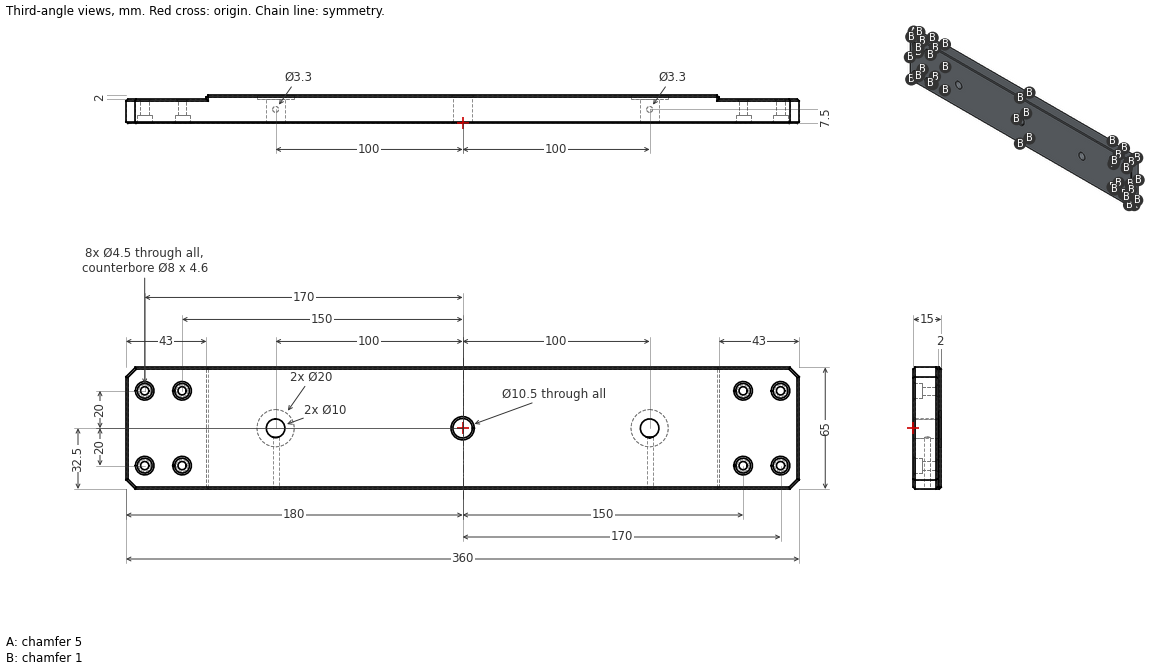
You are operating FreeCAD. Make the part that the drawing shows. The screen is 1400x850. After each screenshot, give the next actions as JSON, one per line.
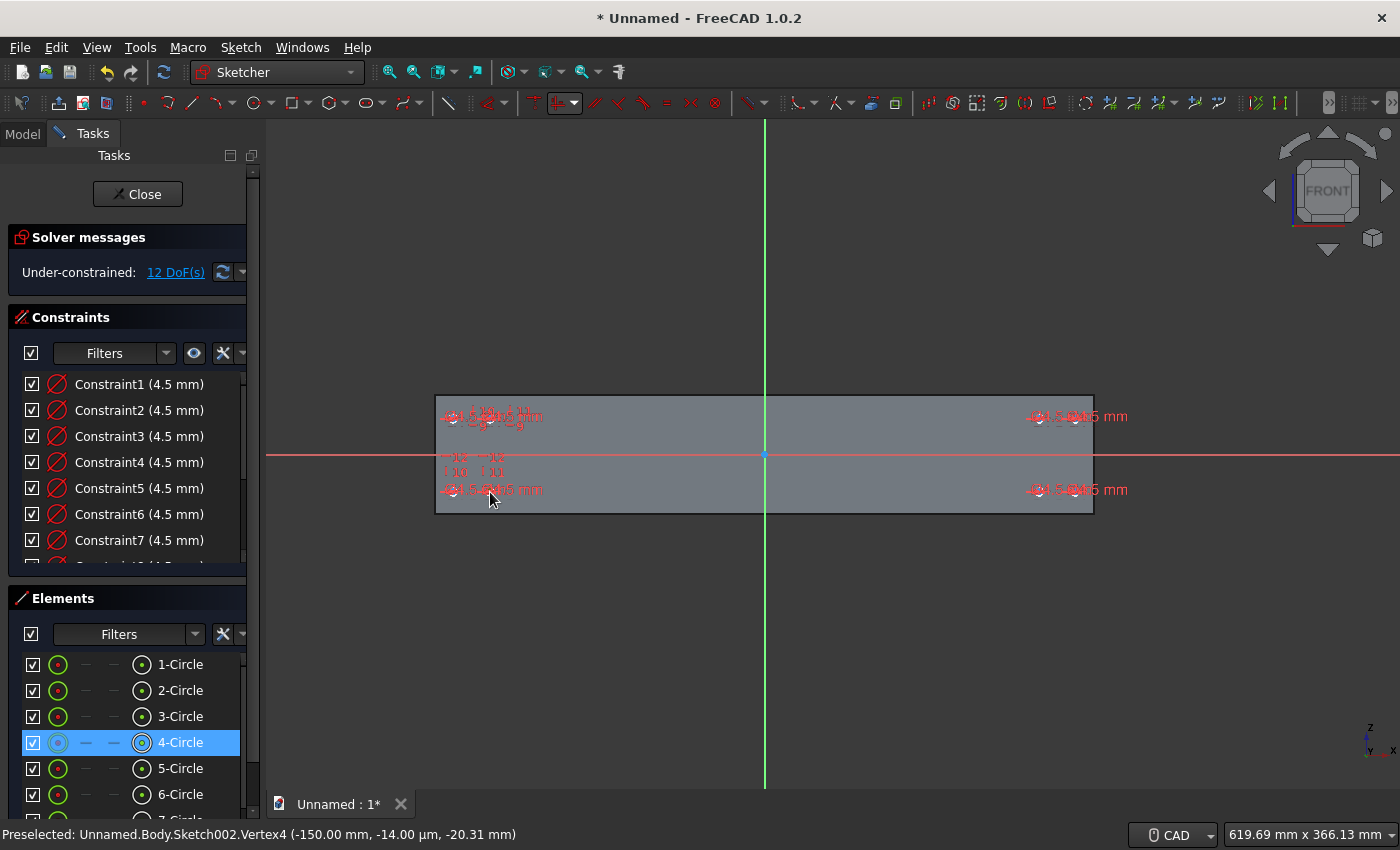
{"action": "left_click", "coordinate": [1039, 492]}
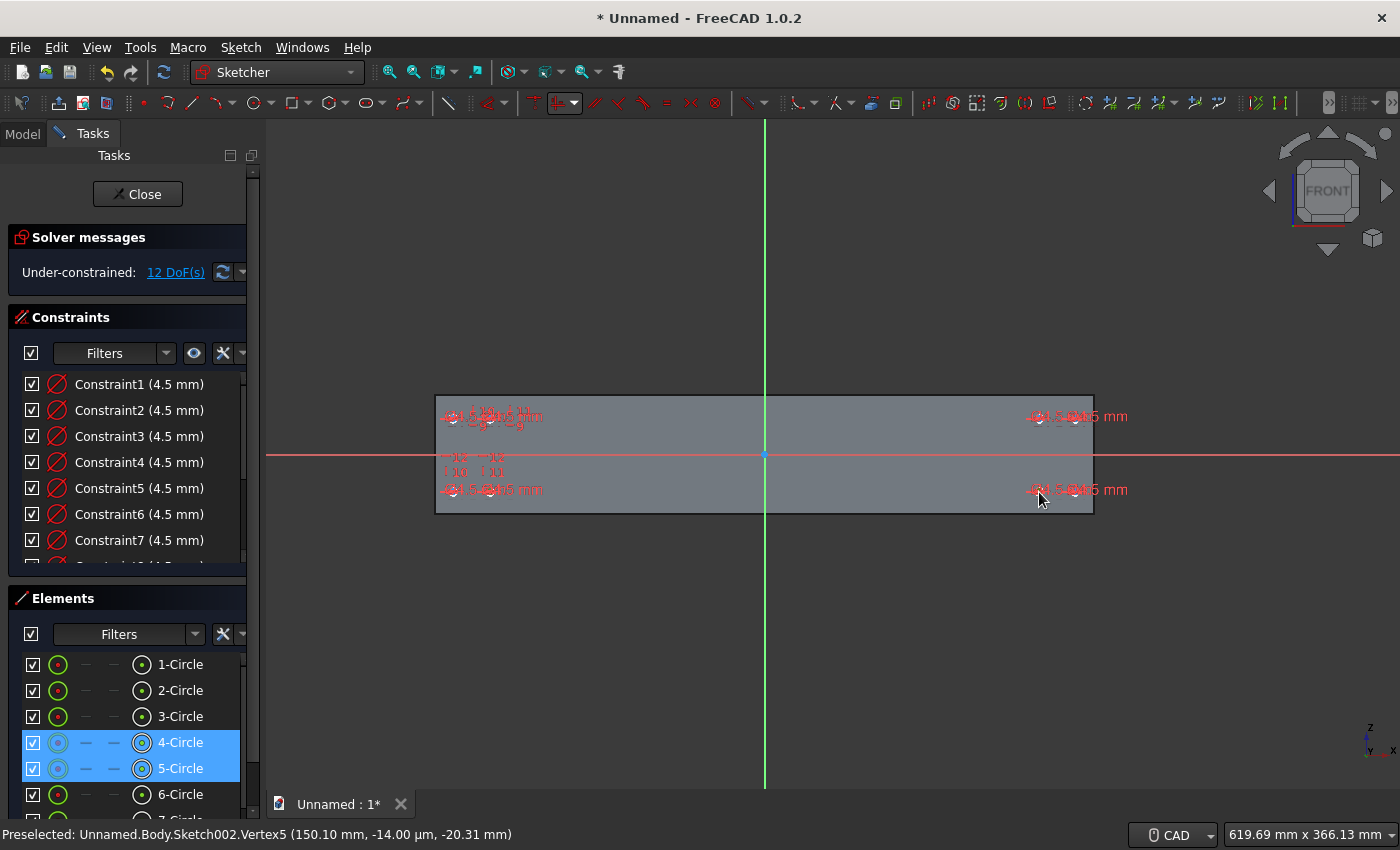
{"action": "left_click", "coordinate": [576, 104]}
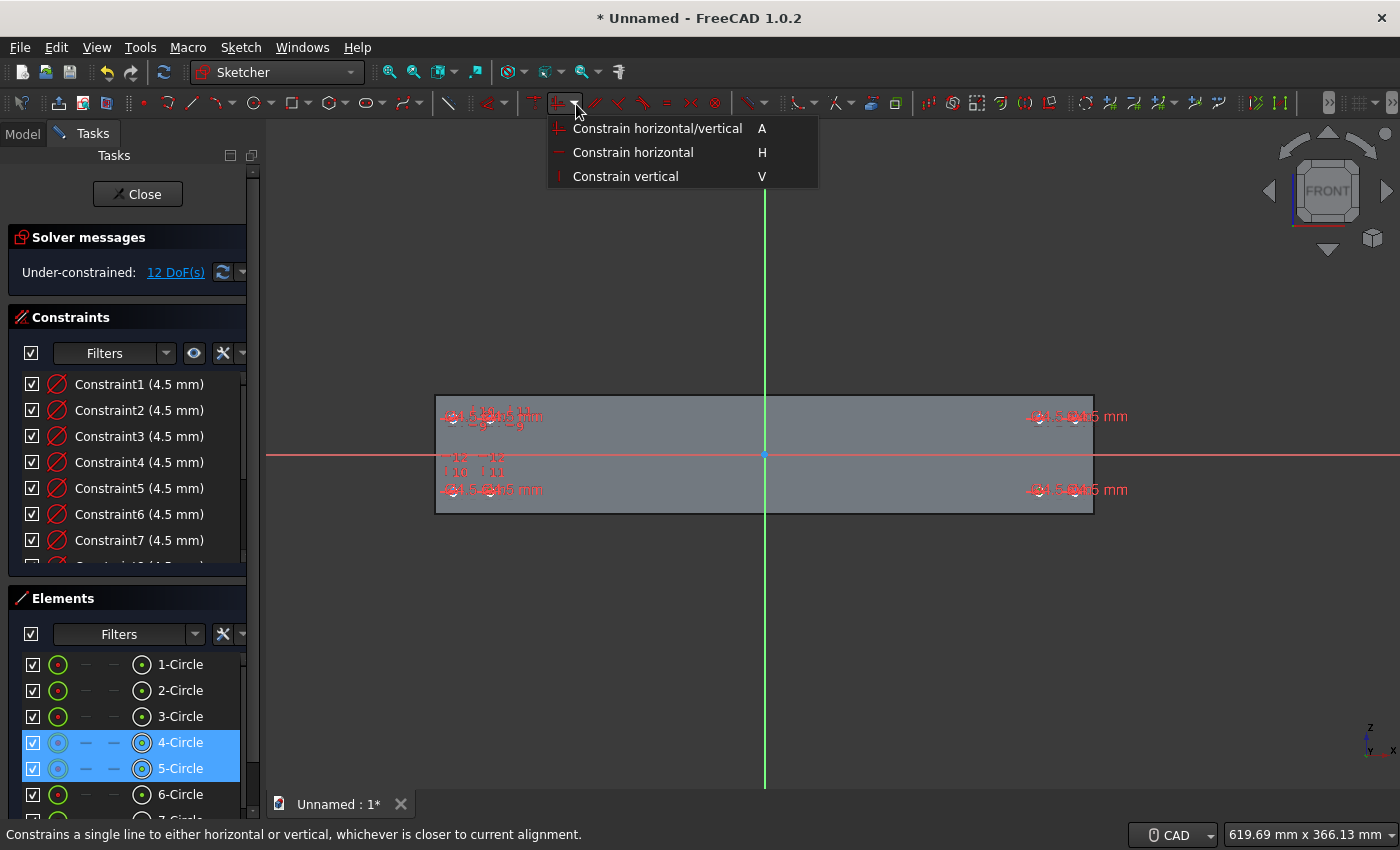
{"action": "left_click", "coordinate": [683, 152]}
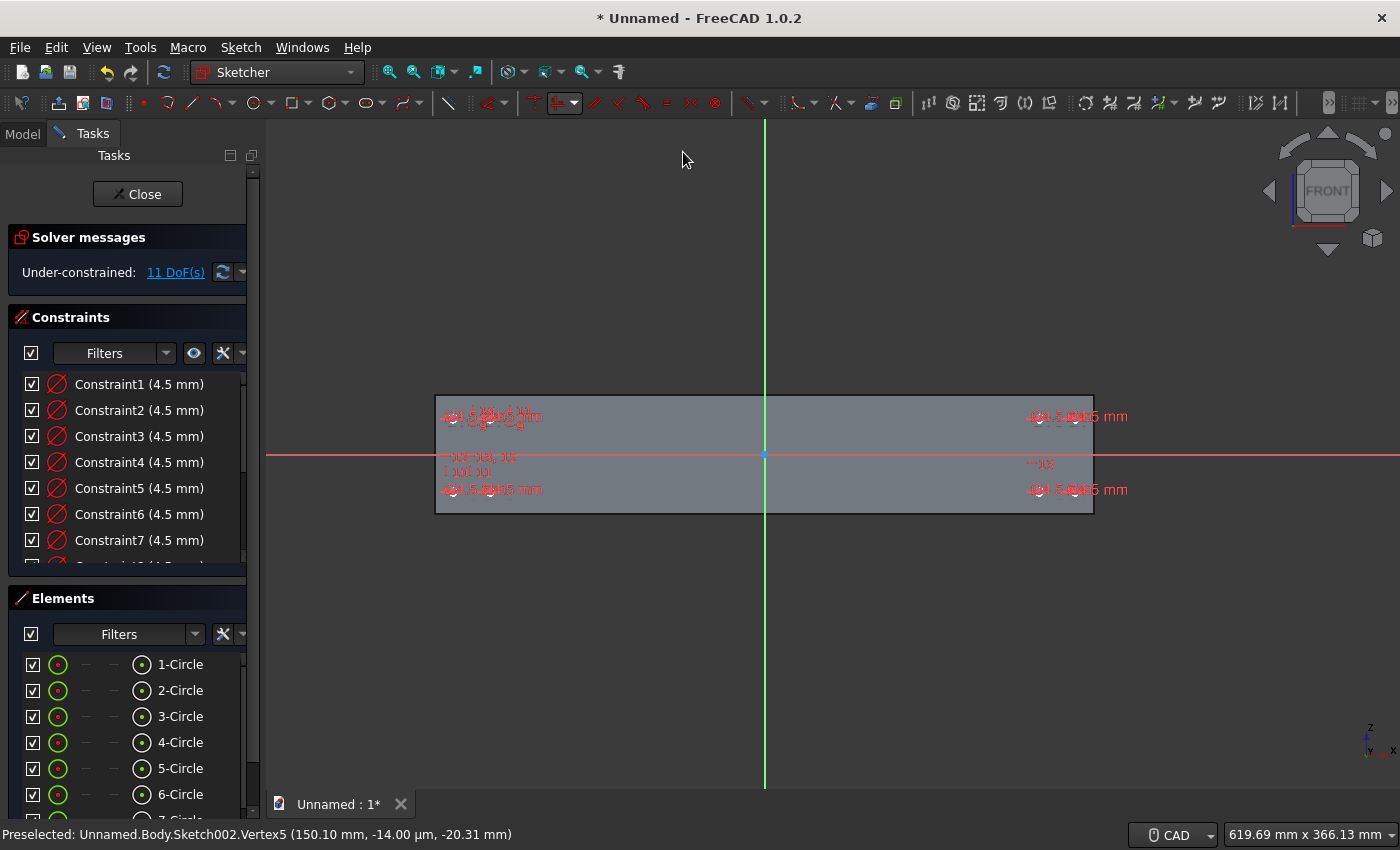
{"action": "left_click", "coordinate": [1039, 492]}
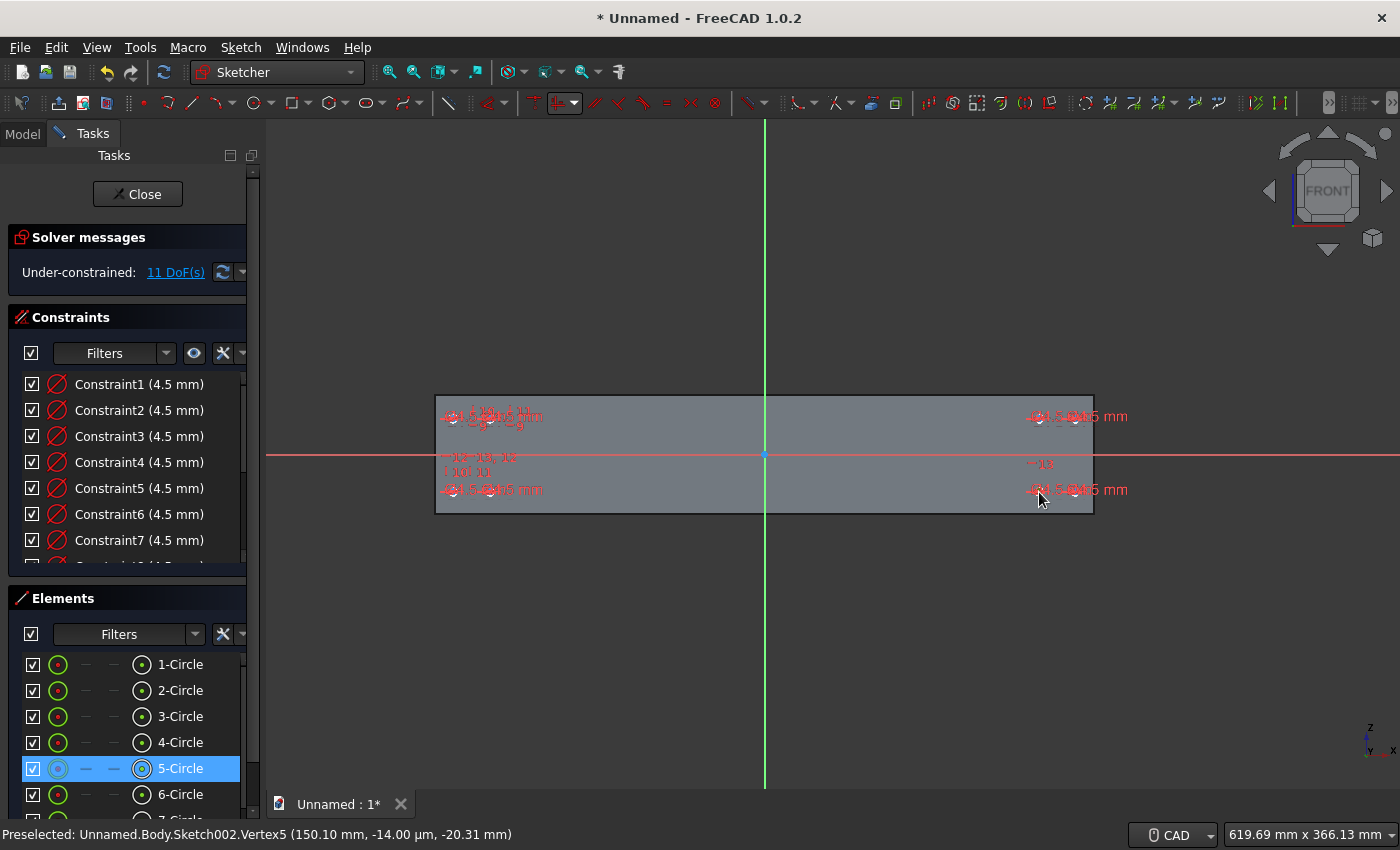
{"action": "left_click", "coordinate": [1075, 492]}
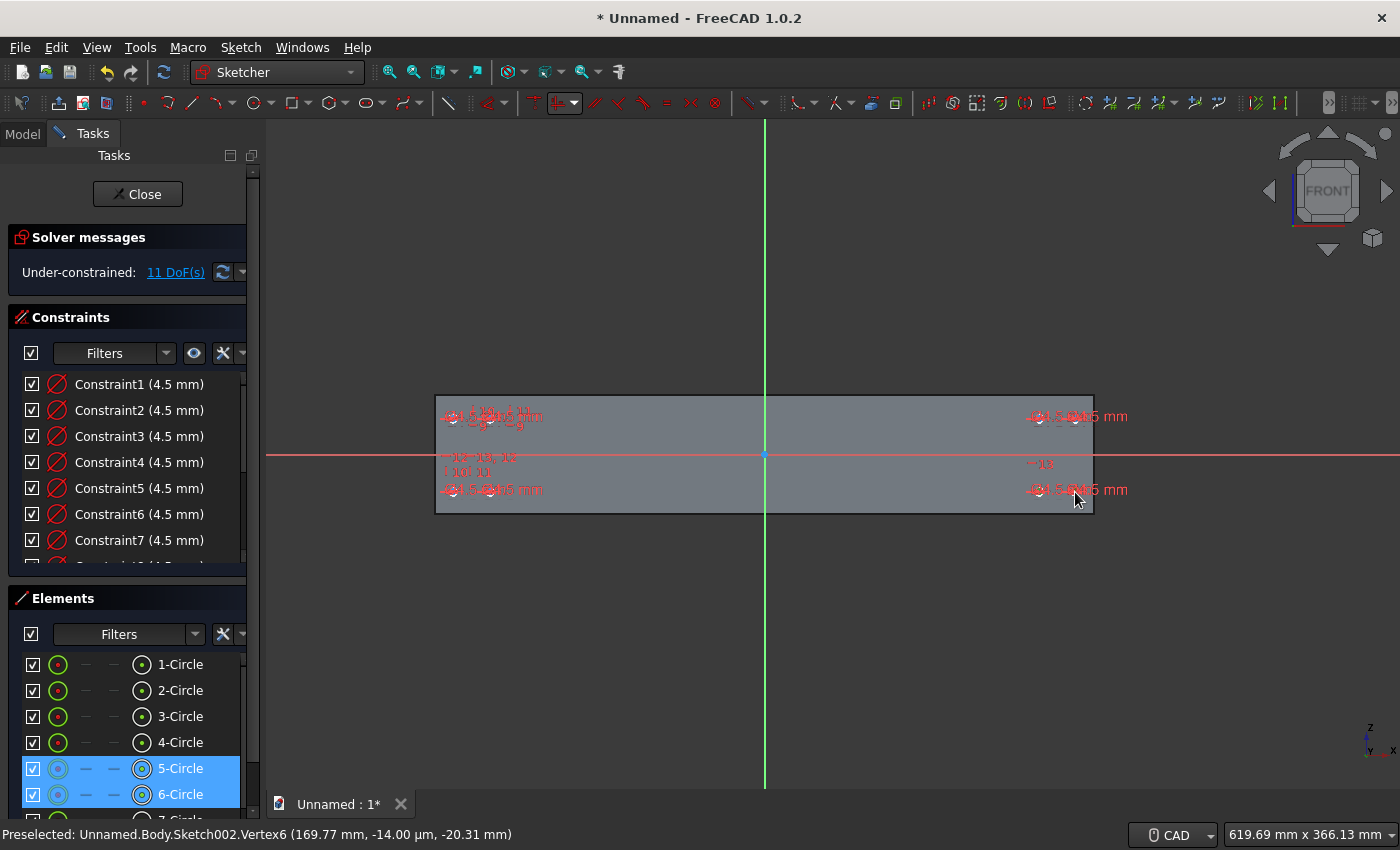
{"action": "left_click", "coordinate": [576, 104]}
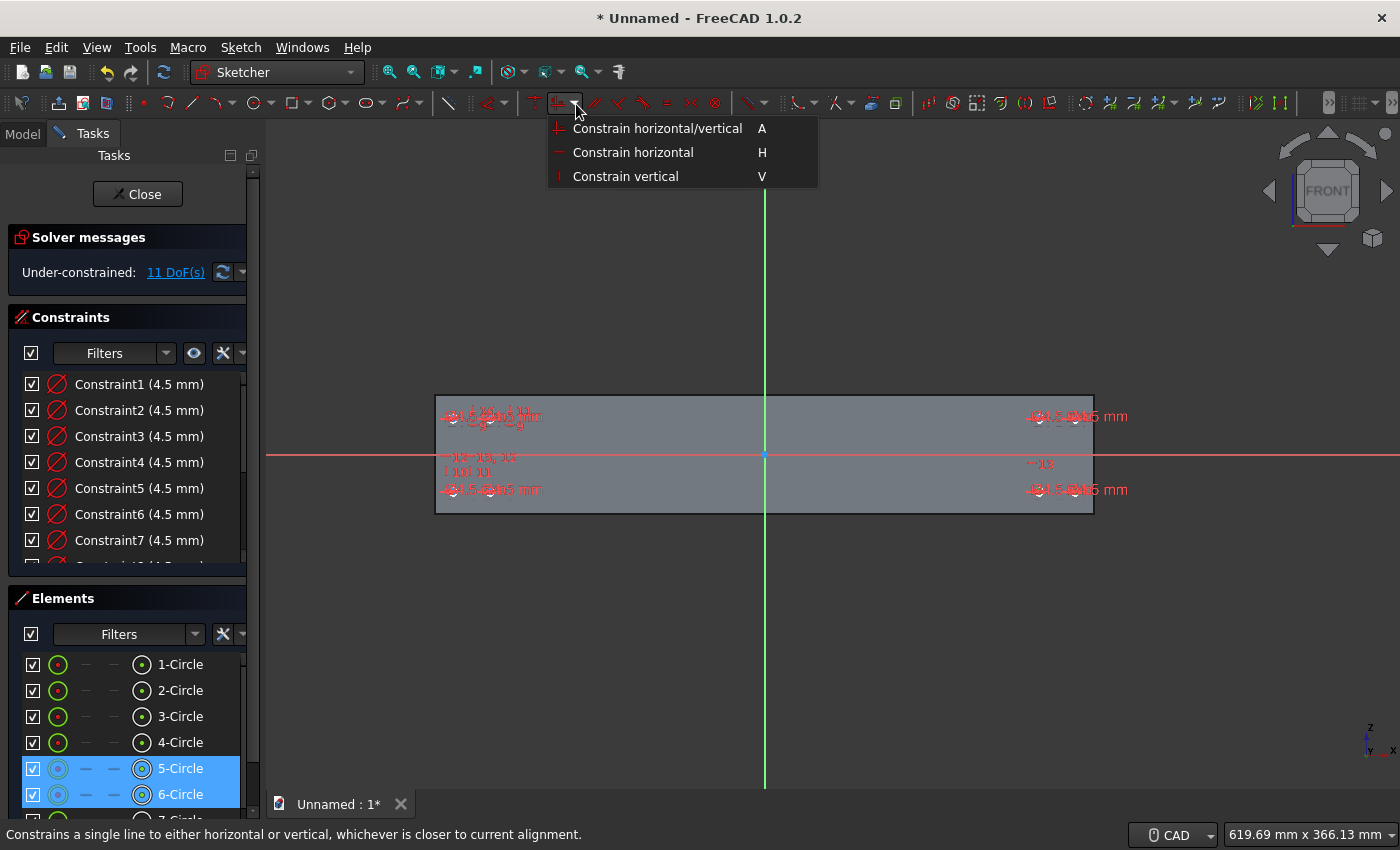
{"action": "left_click", "coordinate": [683, 152]}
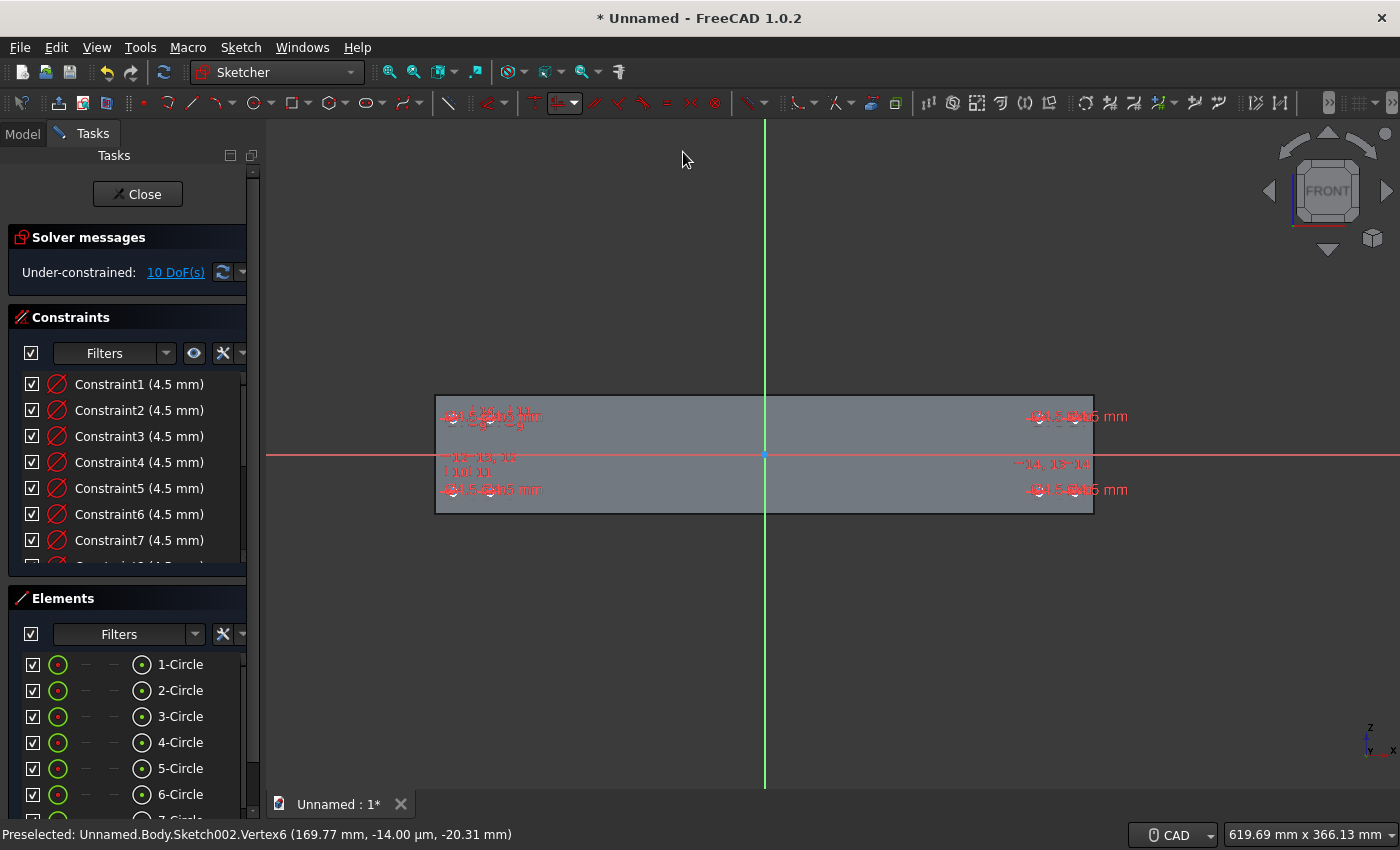
{"action": "left_click", "coordinate": [1039, 492]}